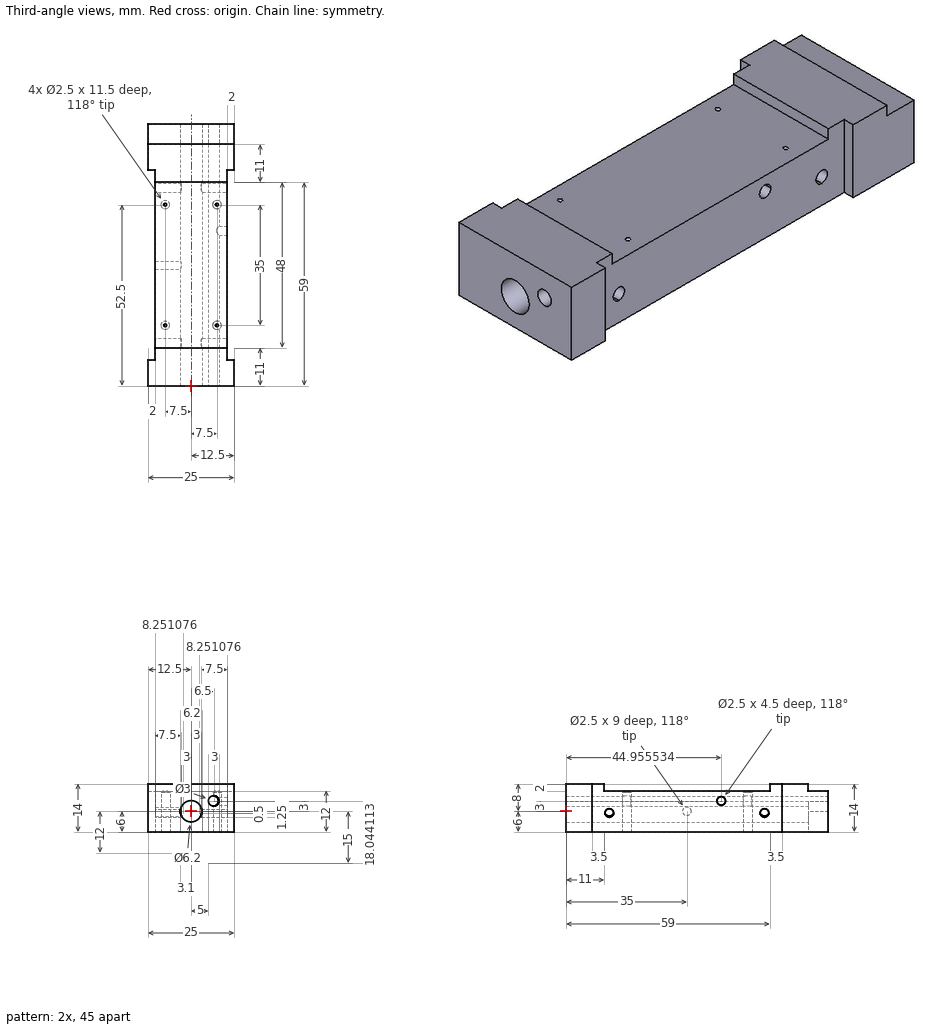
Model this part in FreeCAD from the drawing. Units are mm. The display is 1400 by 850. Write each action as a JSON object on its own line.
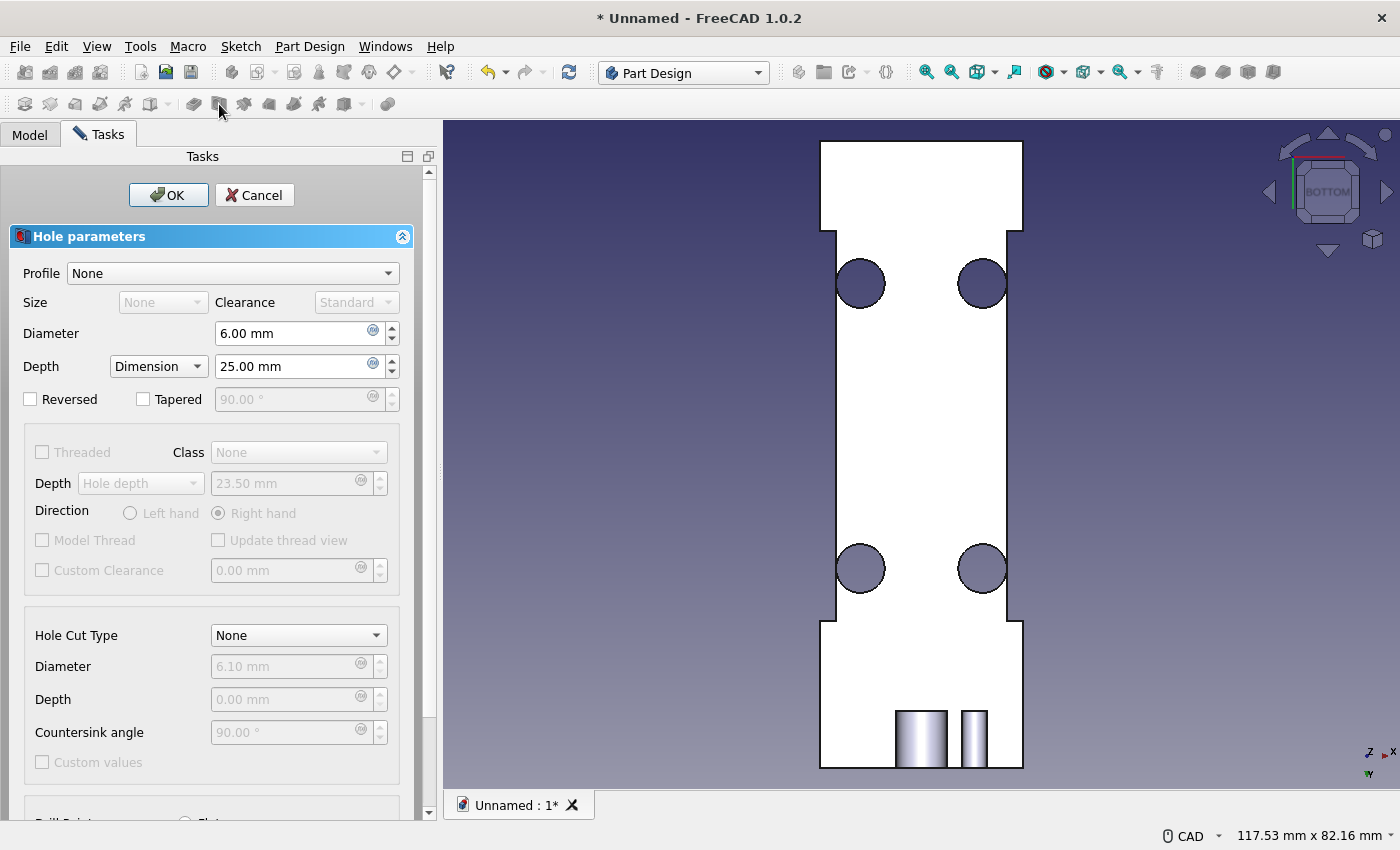
{"action": "triple_click", "coordinate": [300, 334]}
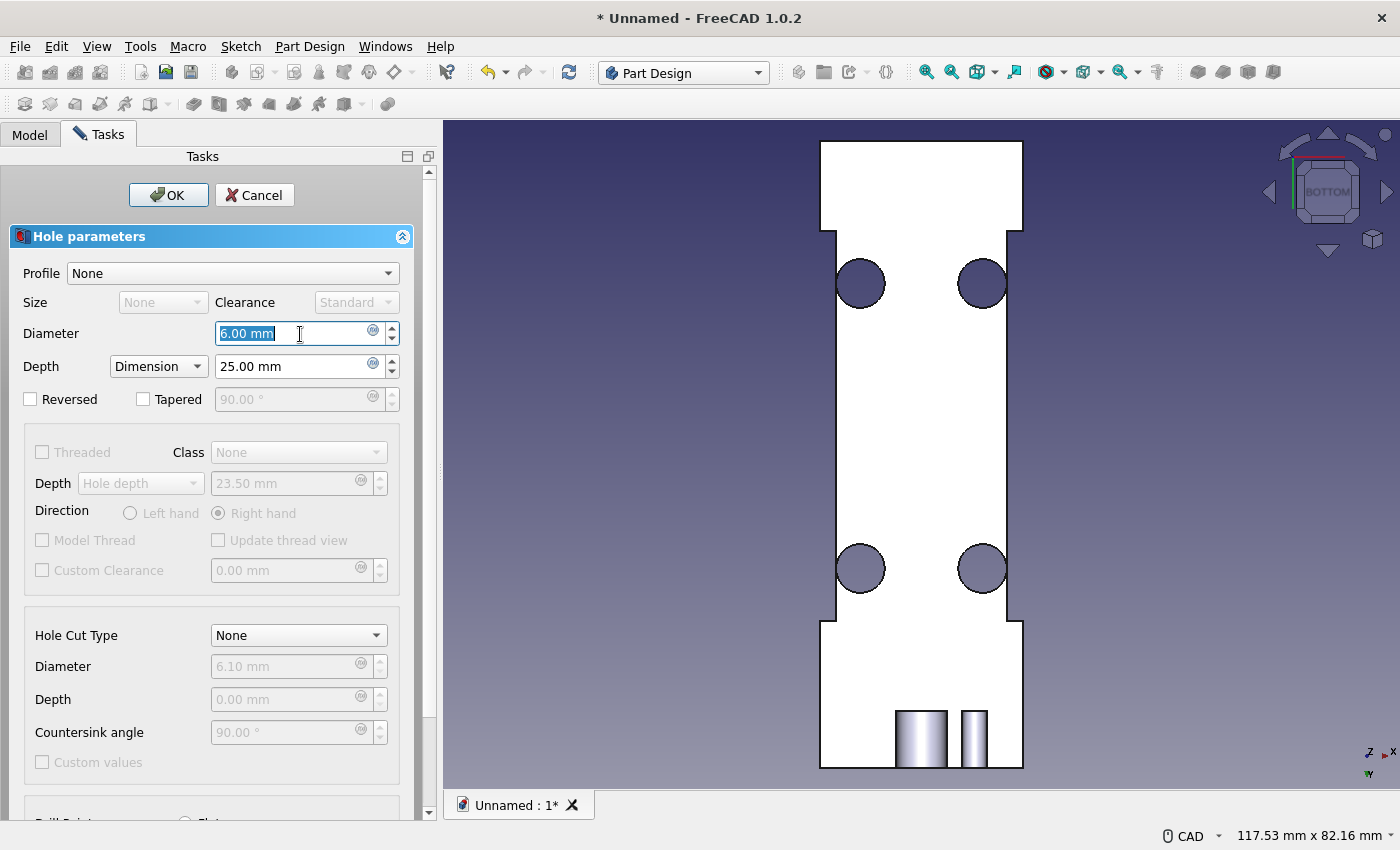
{"action": "type", "text": "2.5"}
{"action": "key", "text": "Tab"}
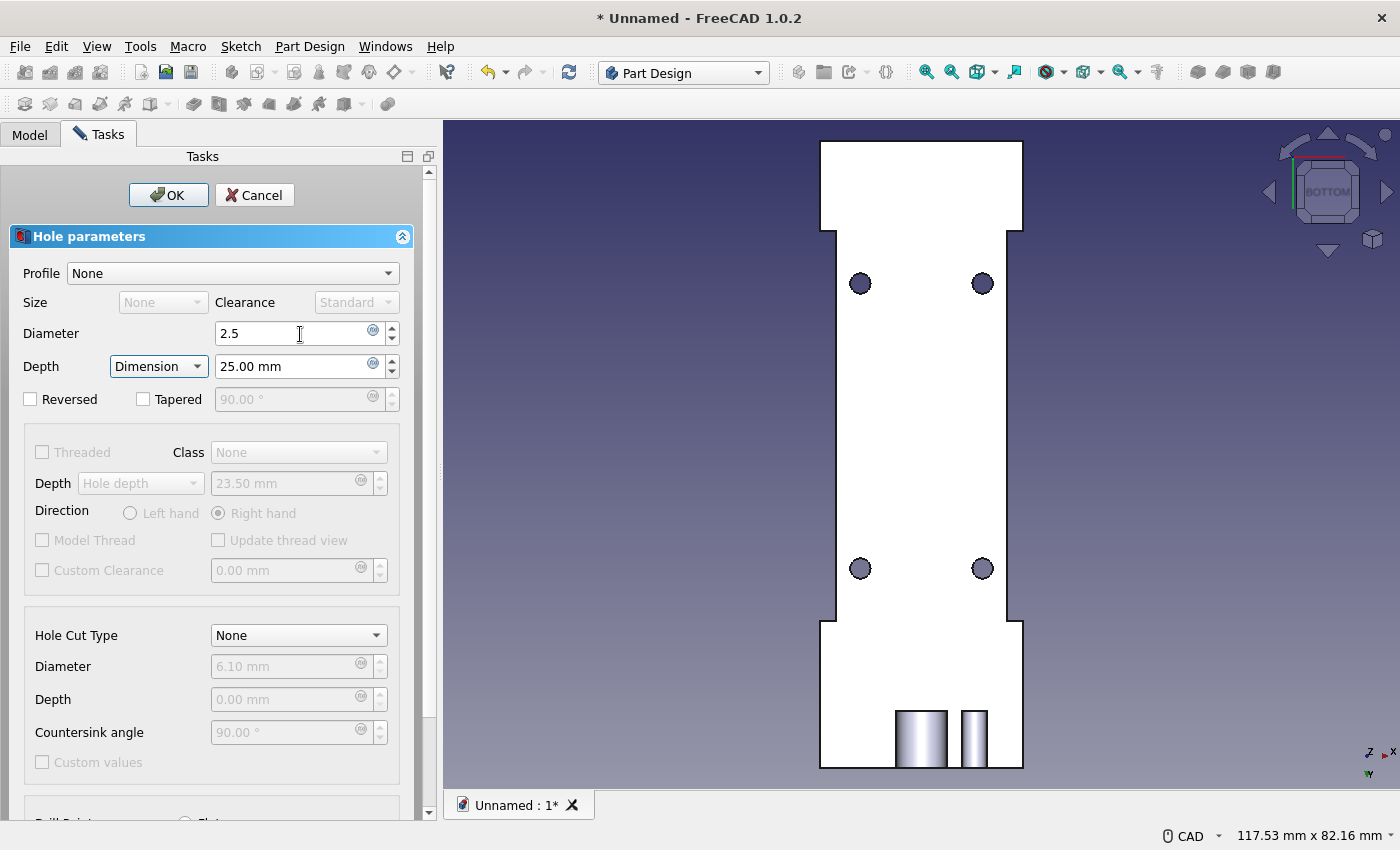
{"action": "triple_click", "coordinate": [300, 366]}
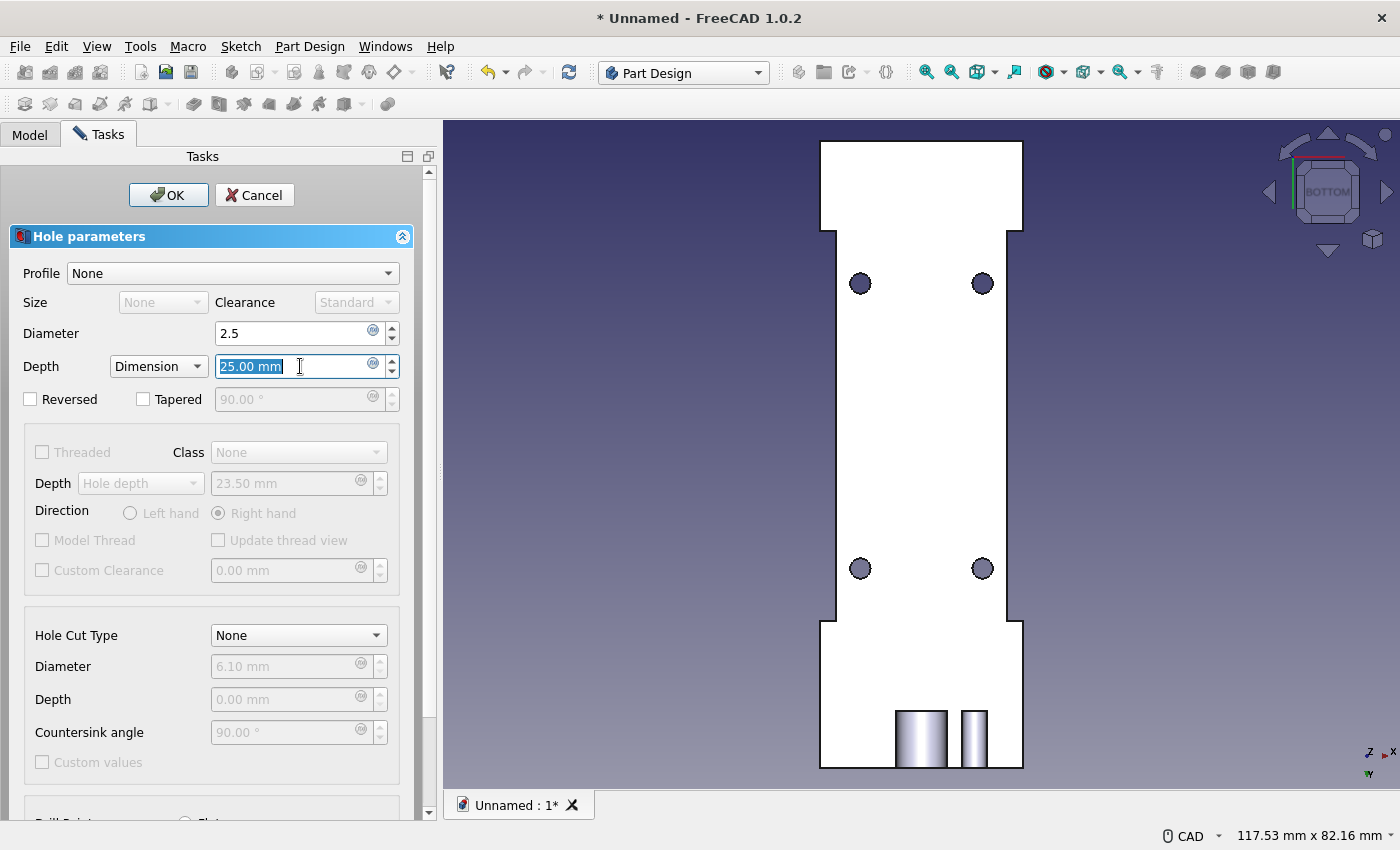
{"action": "type", "text": "11.5"}
{"action": "key", "text": "Tab"}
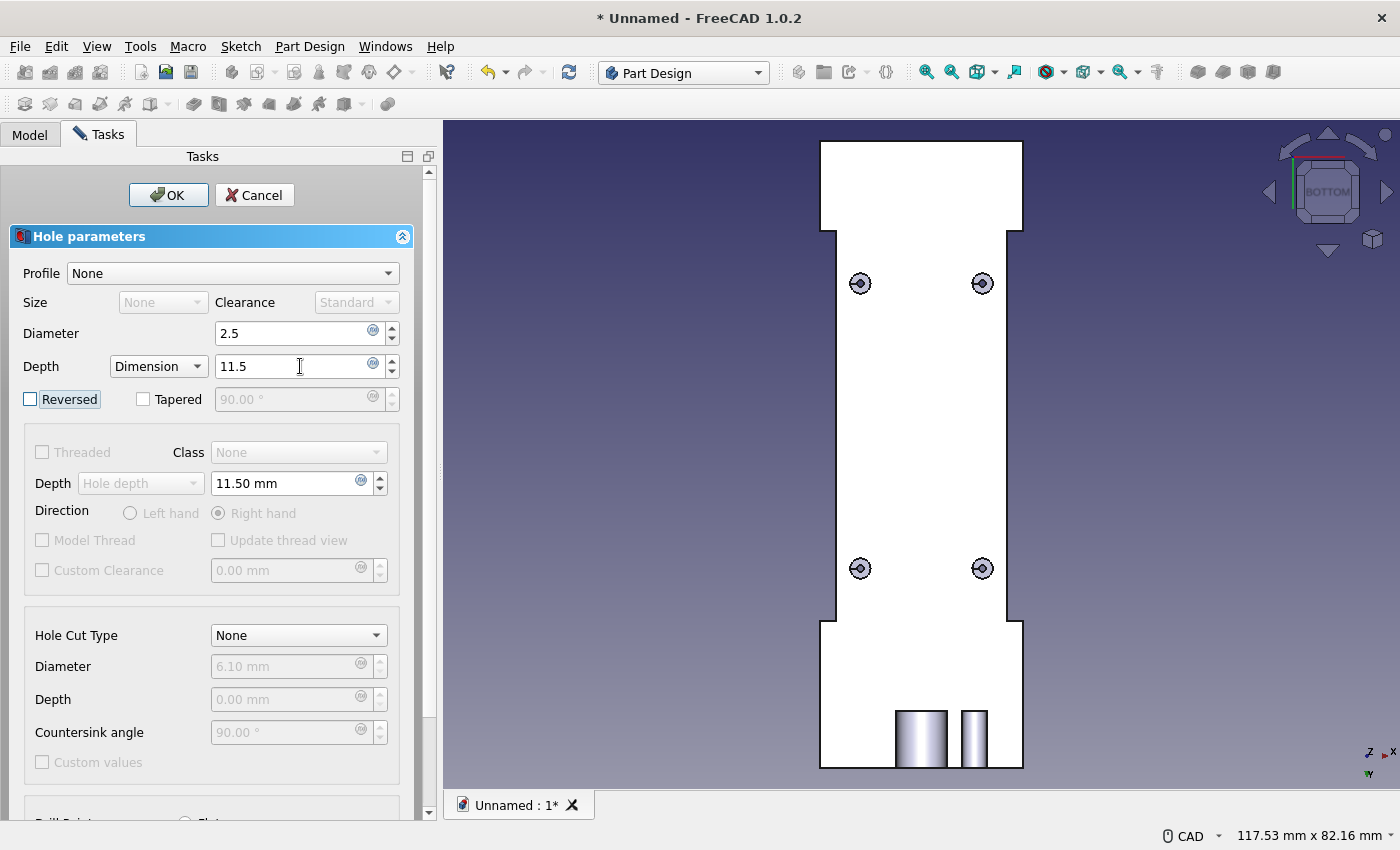
{"action": "left_click", "coordinate": [169, 195]}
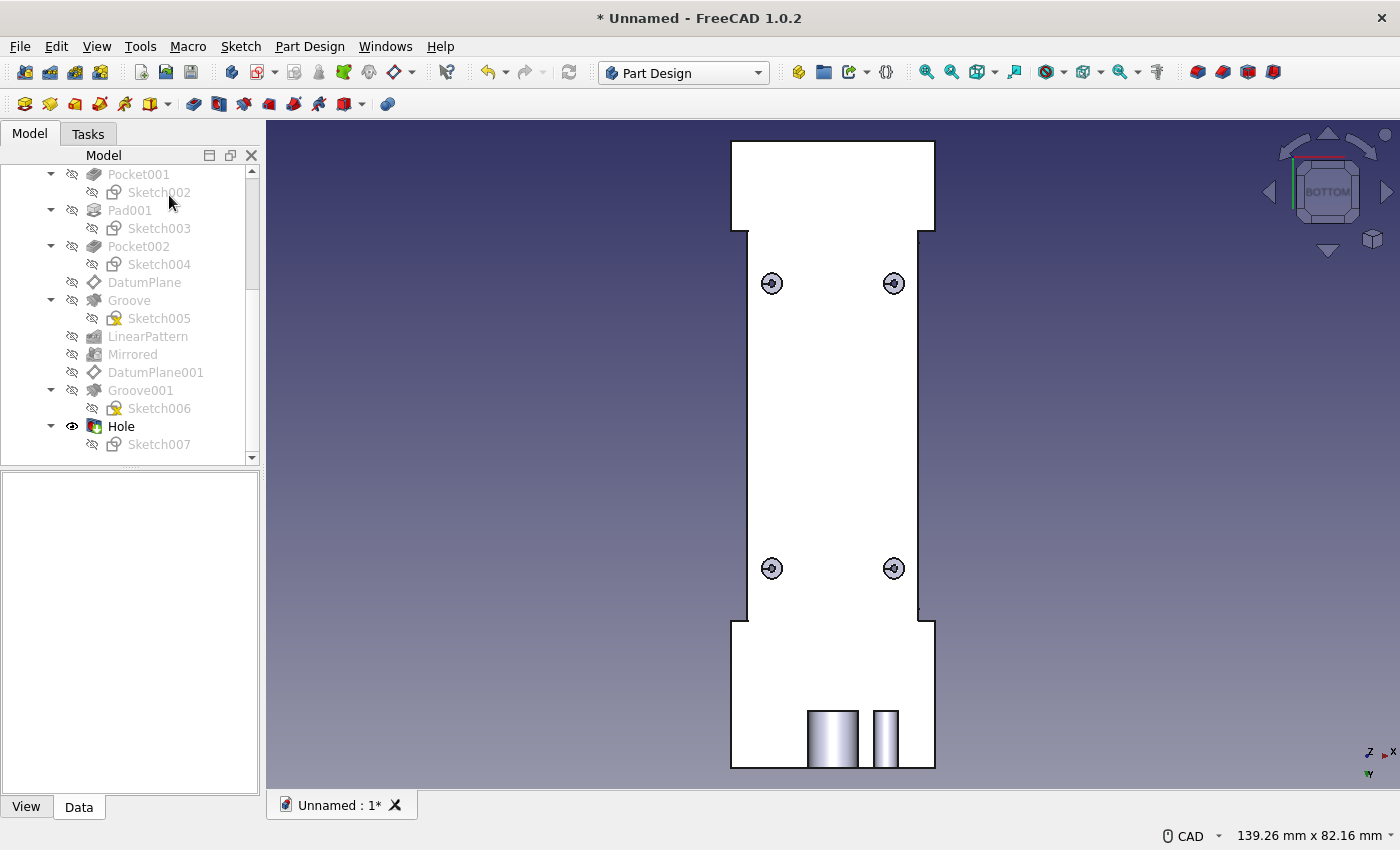
{"action": "key", "text": "0"}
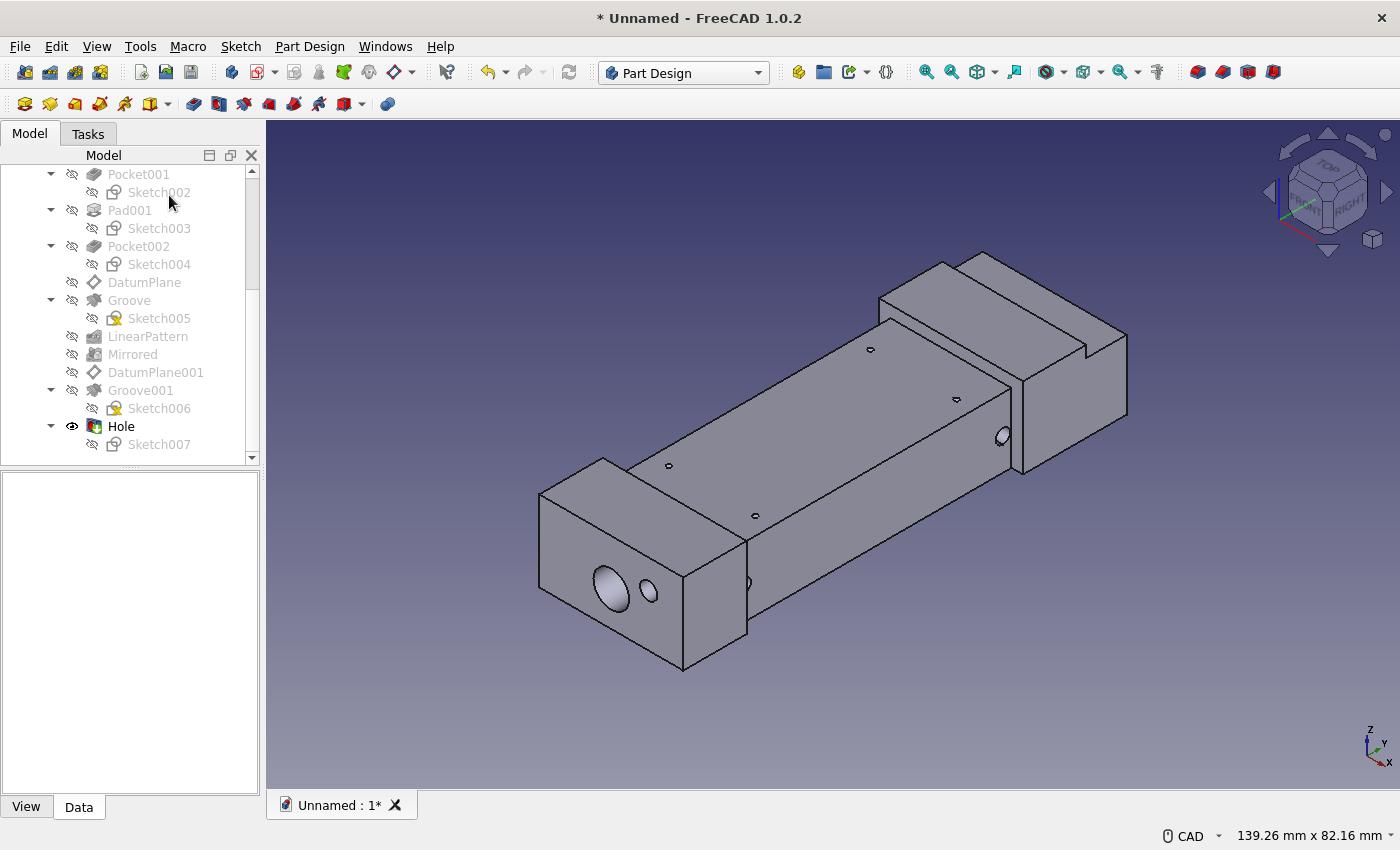
{"action": "left_click", "coordinate": [1060, 406]}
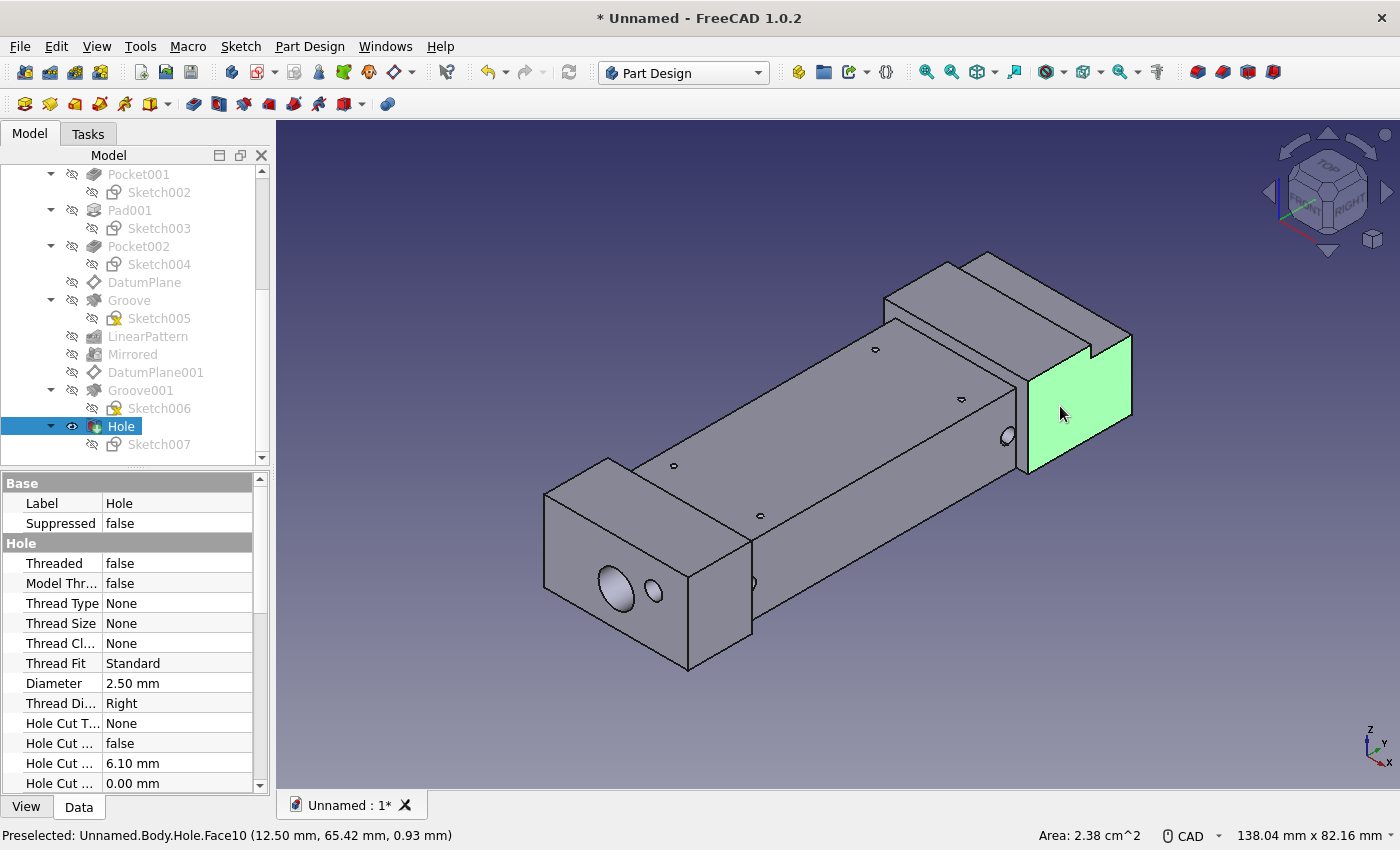
{"action": "left_click", "coordinate": [256, 72]}